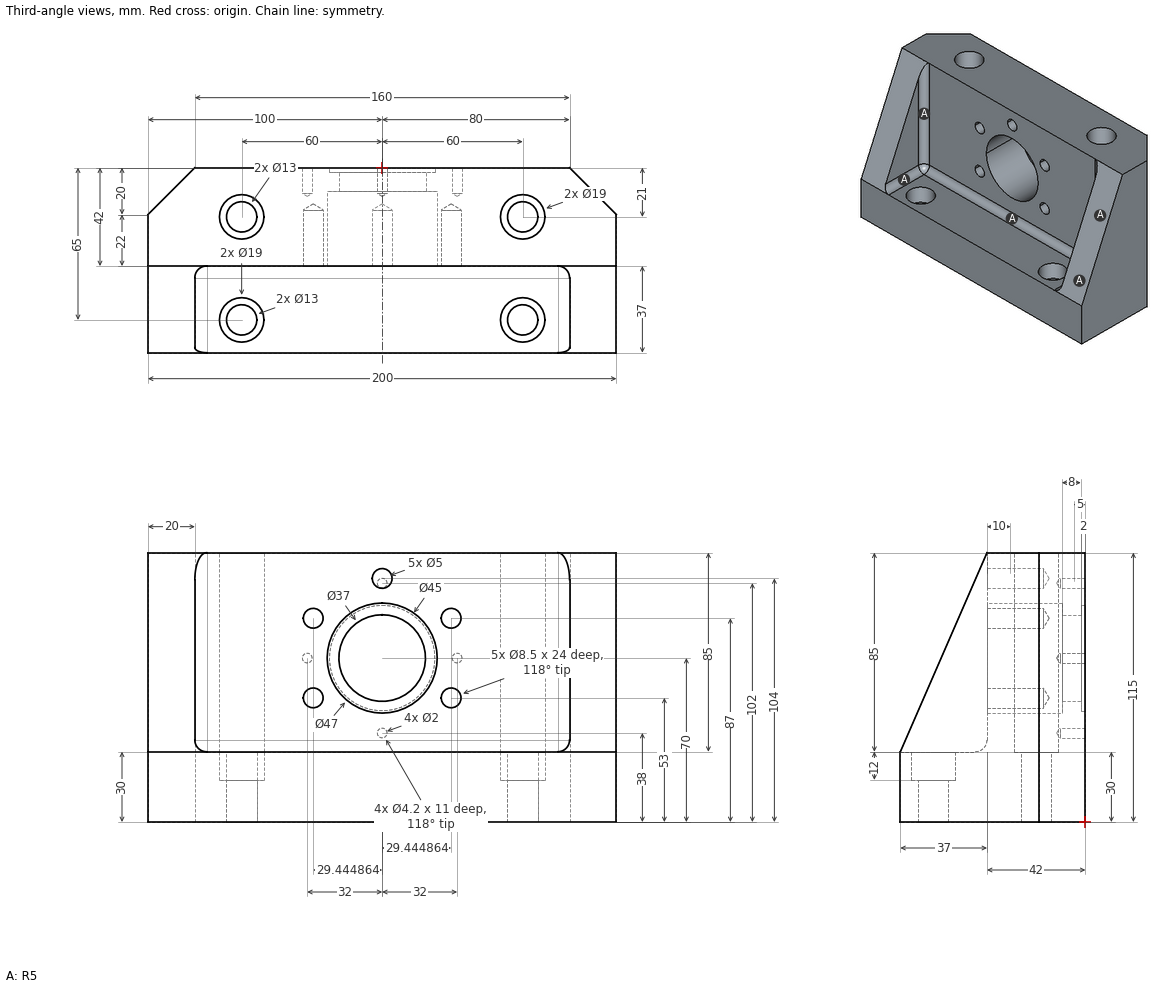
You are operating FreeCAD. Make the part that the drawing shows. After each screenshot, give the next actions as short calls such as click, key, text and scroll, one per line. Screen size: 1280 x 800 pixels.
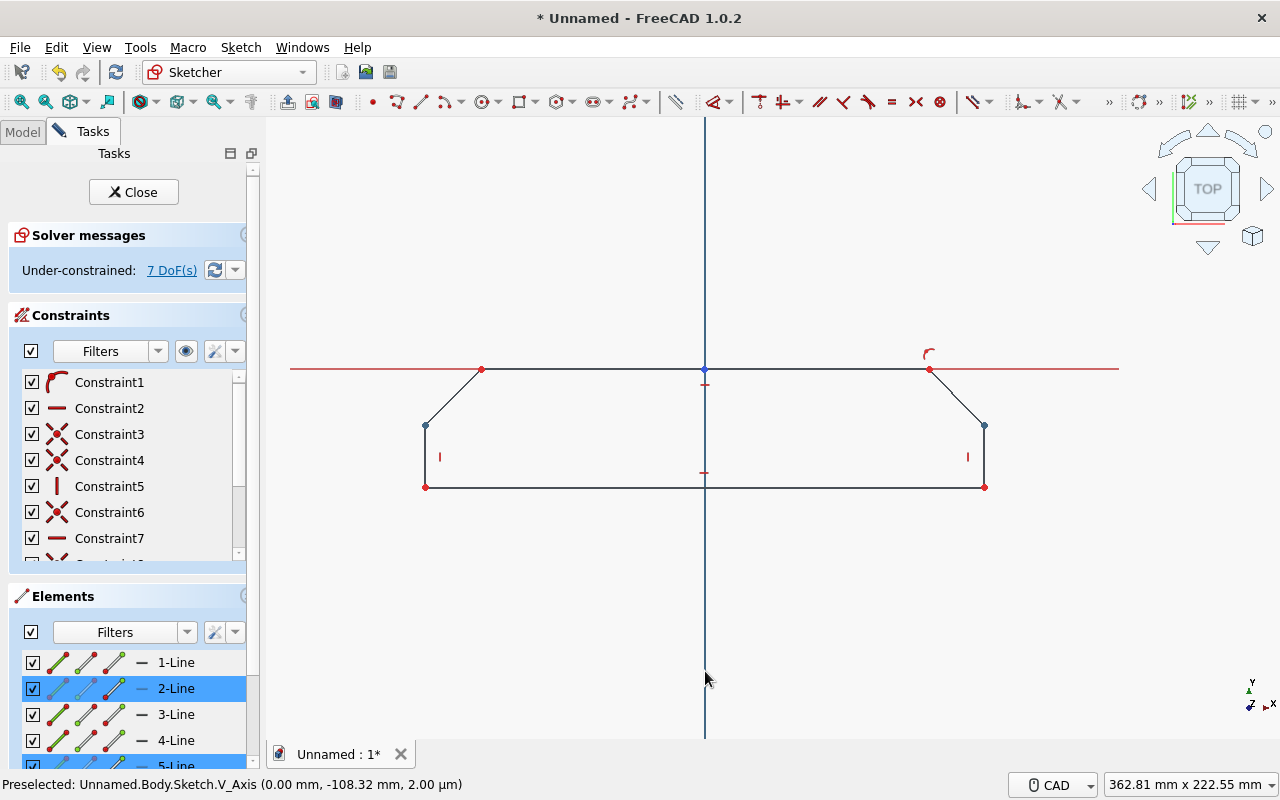
key(s)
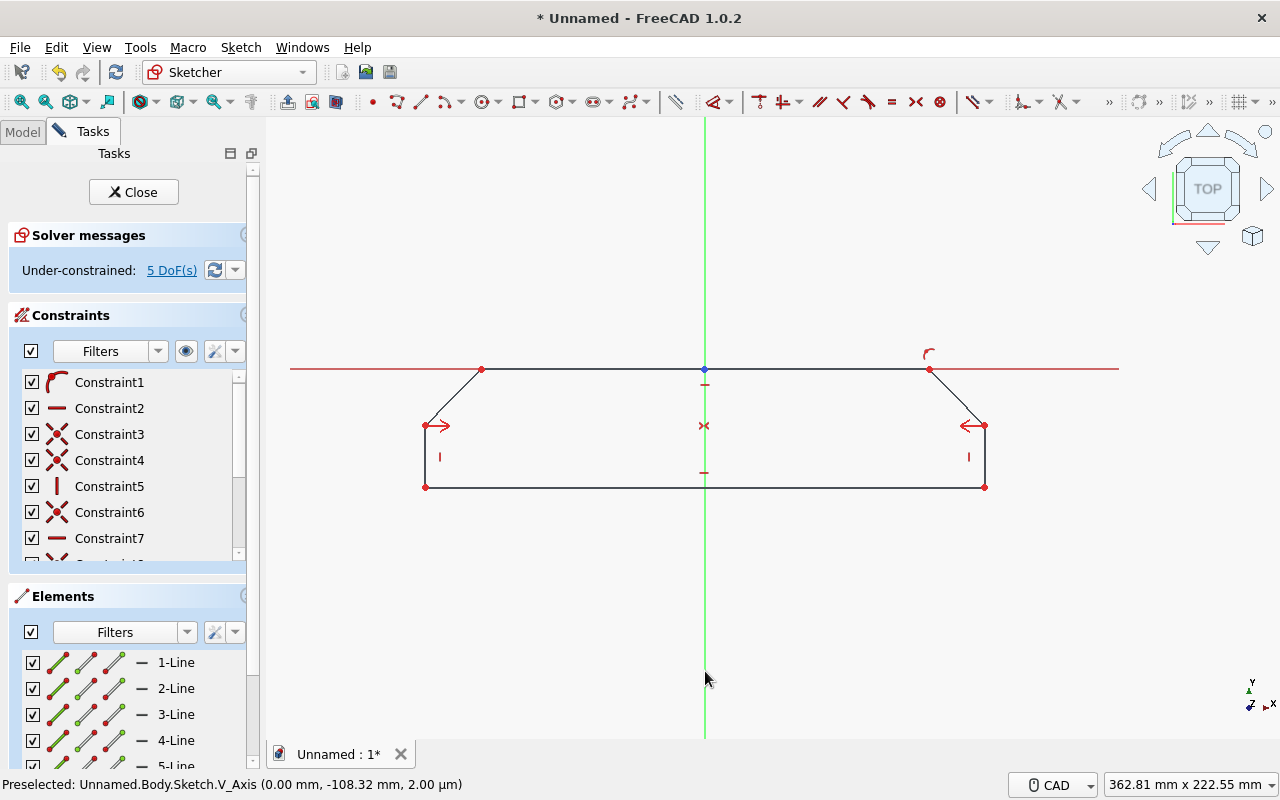
click(714, 102)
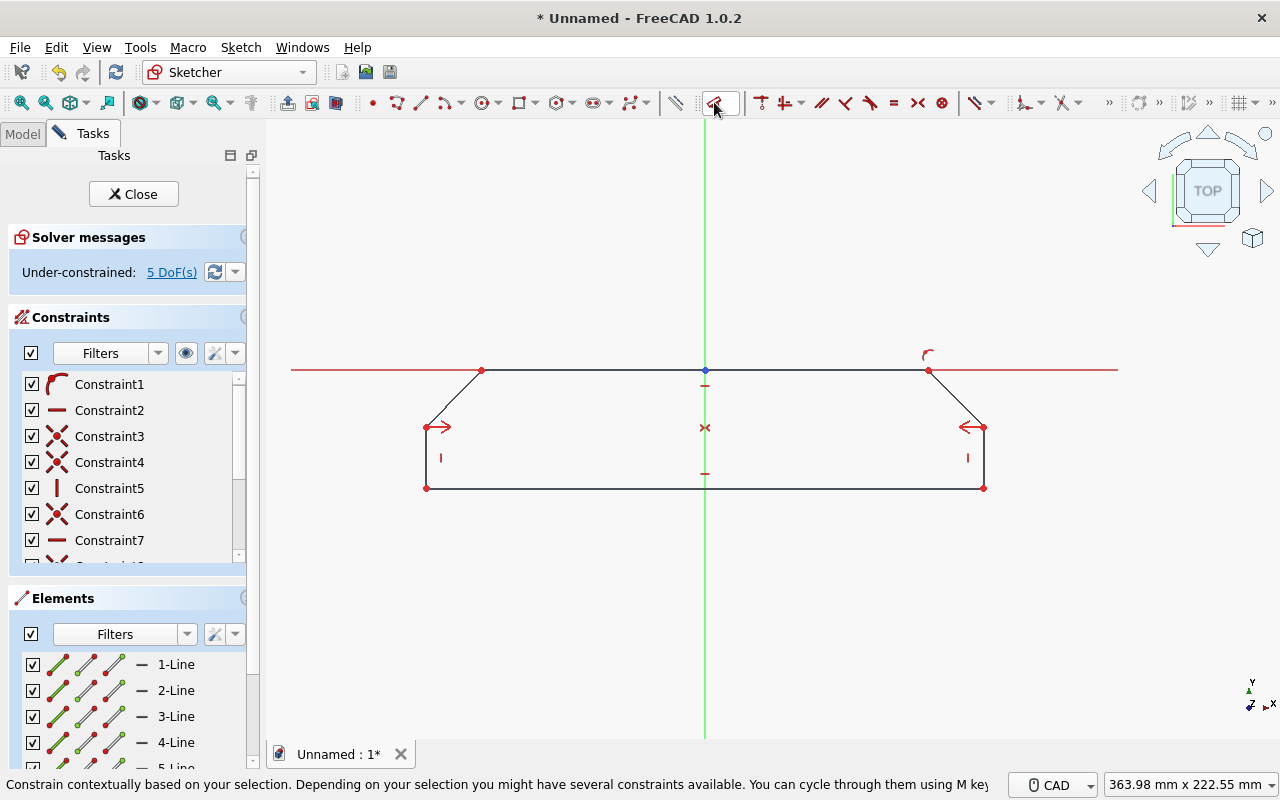
click(426, 446)
click(392, 458)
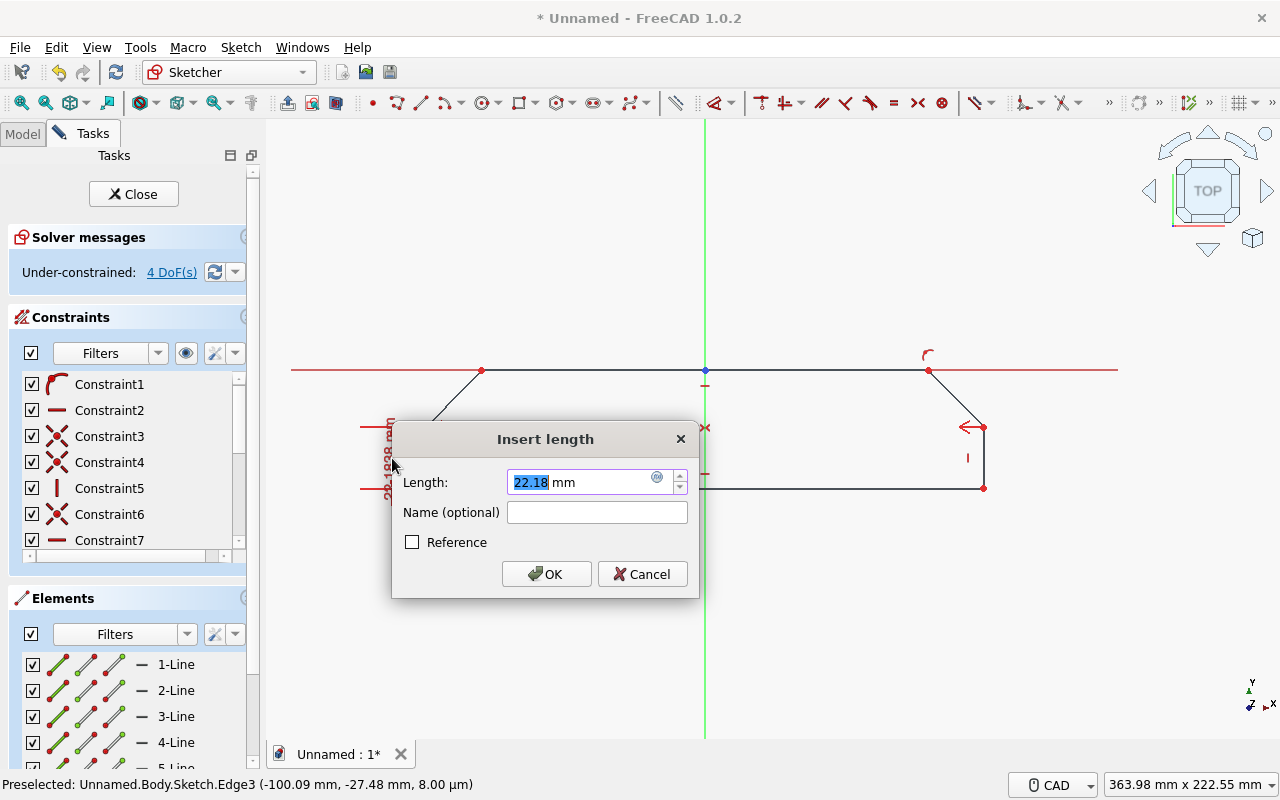
text(22)
key(Return)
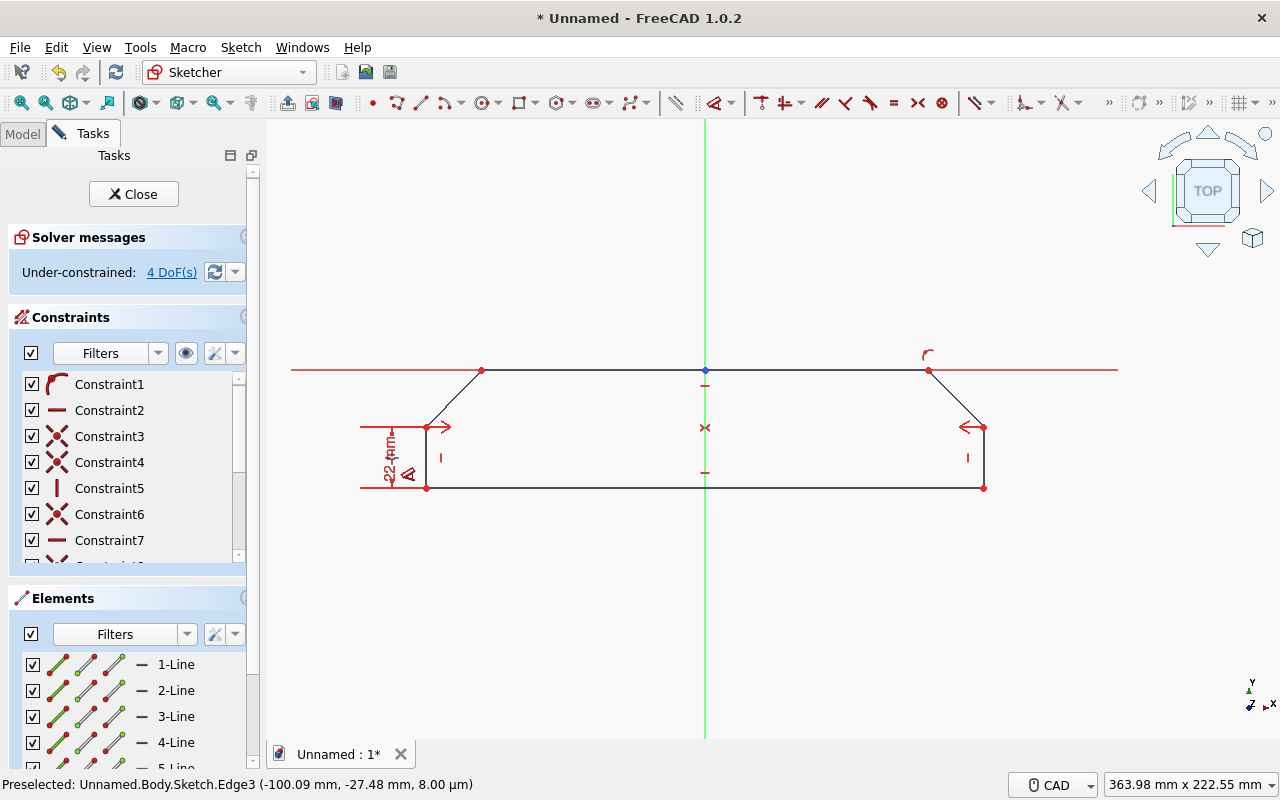
click(795, 370)
click(603, 336)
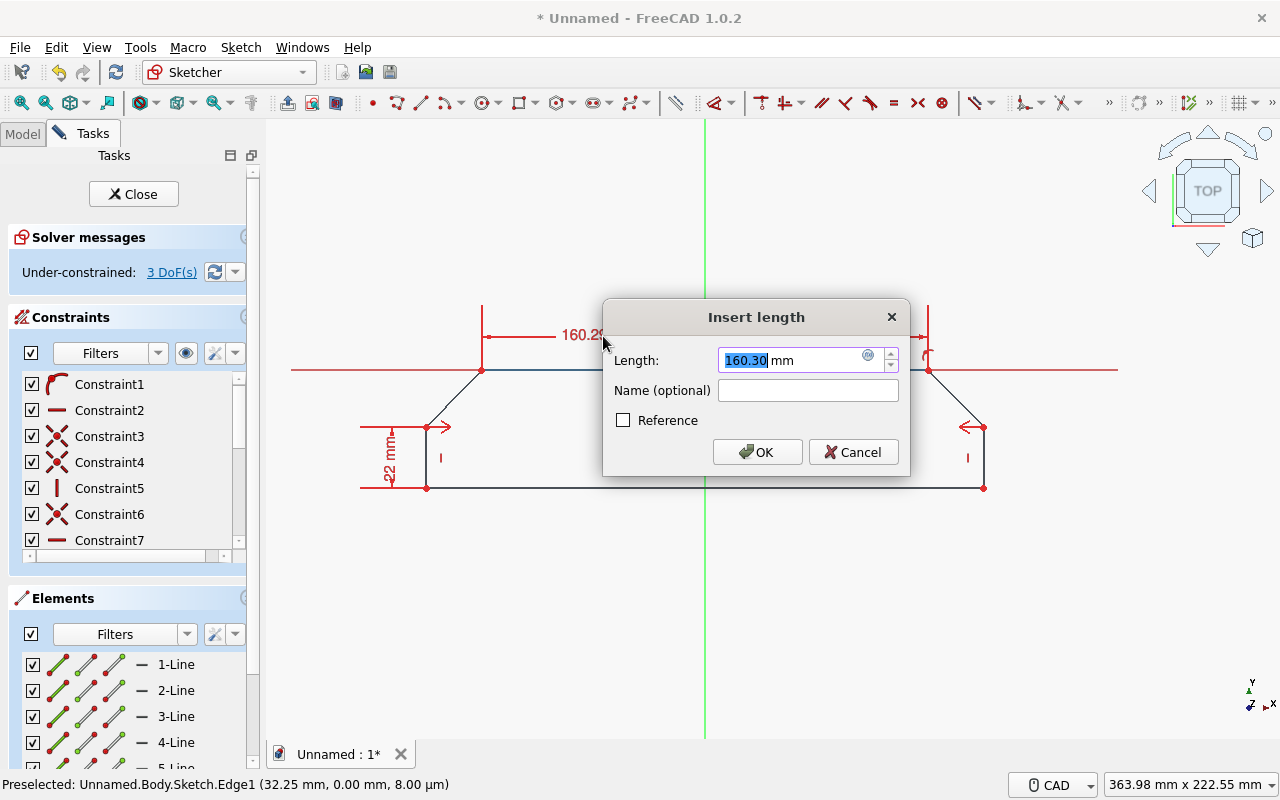
text(160)
key(Return)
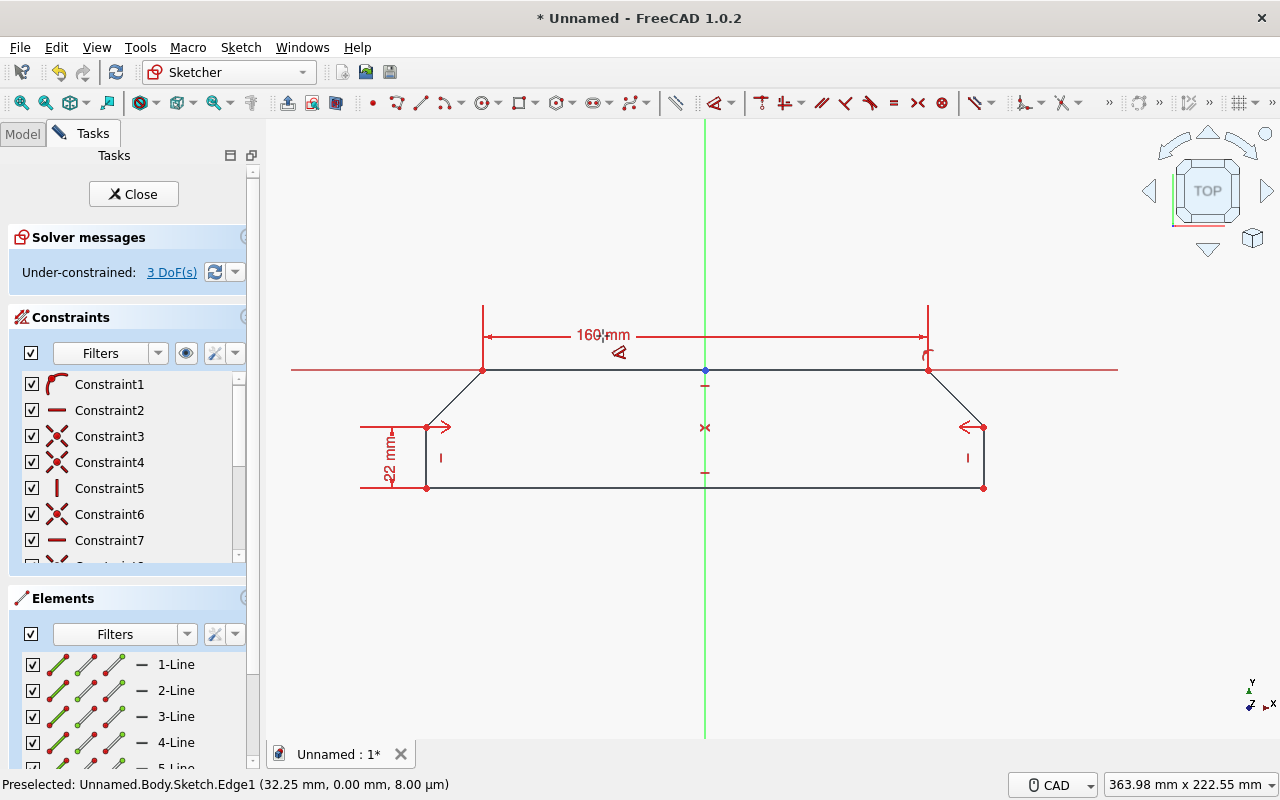
click(594, 488)
click(577, 522)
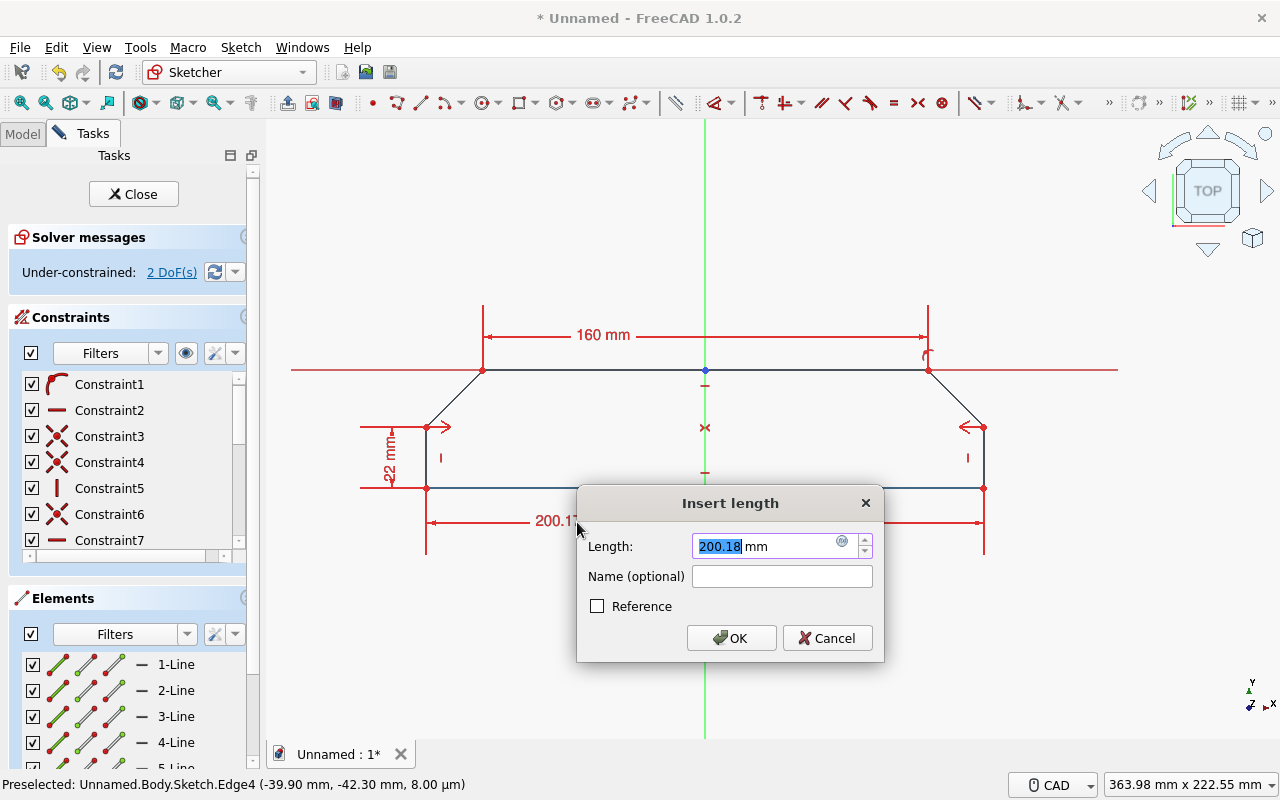
text(200)
key(Return)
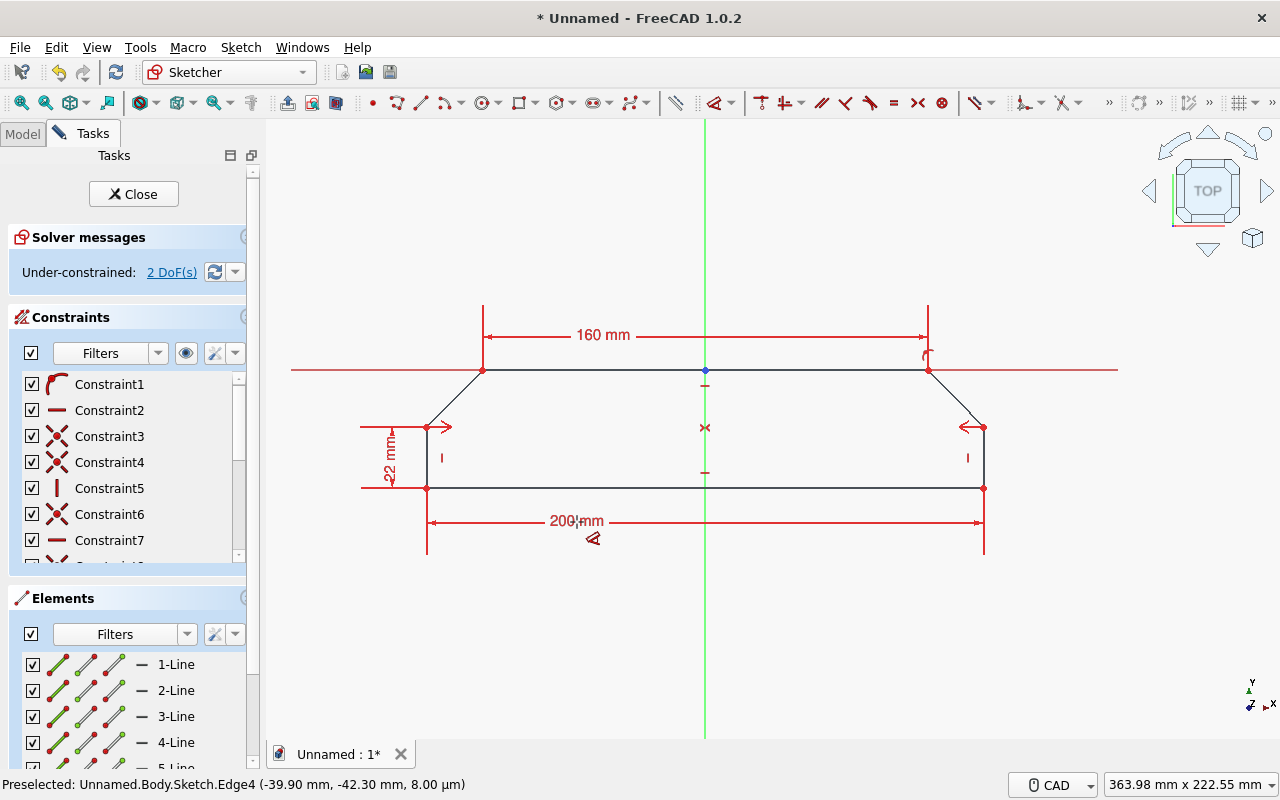
click(928, 370)
click(817, 336)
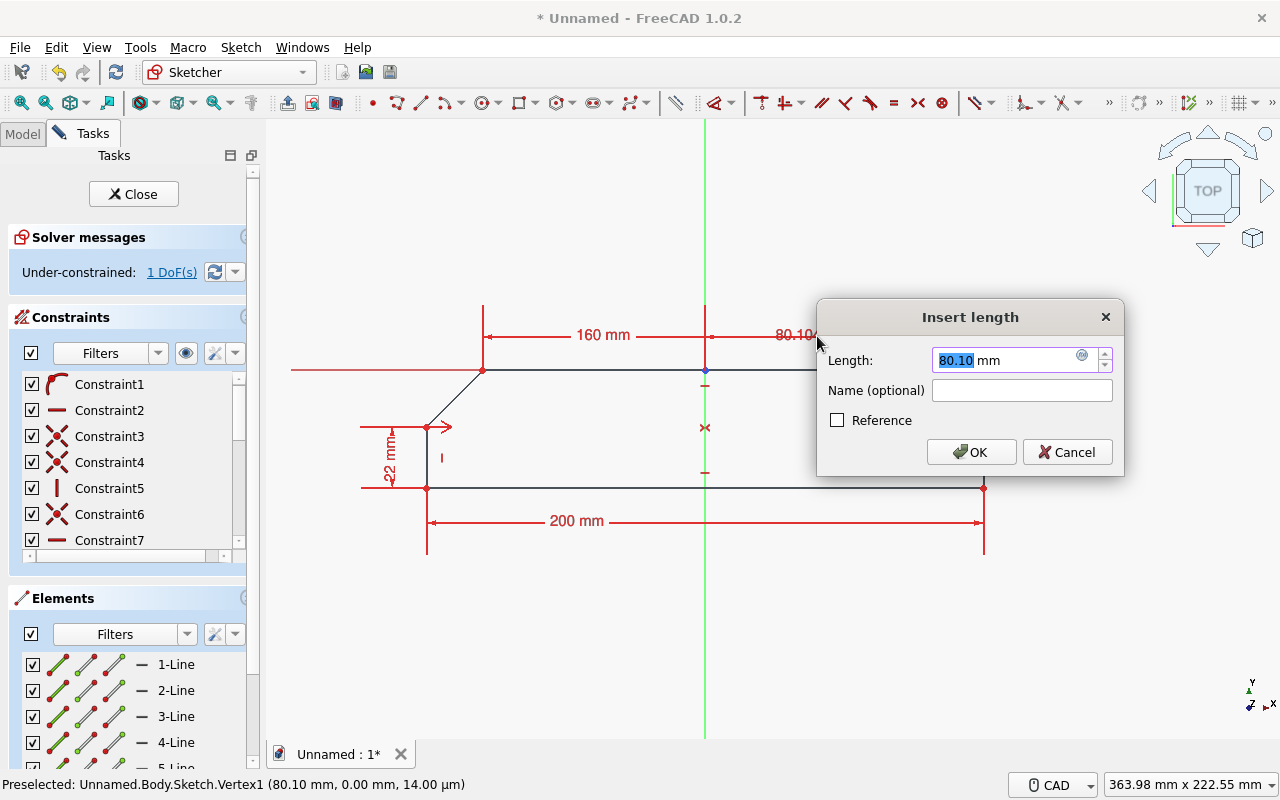
text(80)
key(Return)